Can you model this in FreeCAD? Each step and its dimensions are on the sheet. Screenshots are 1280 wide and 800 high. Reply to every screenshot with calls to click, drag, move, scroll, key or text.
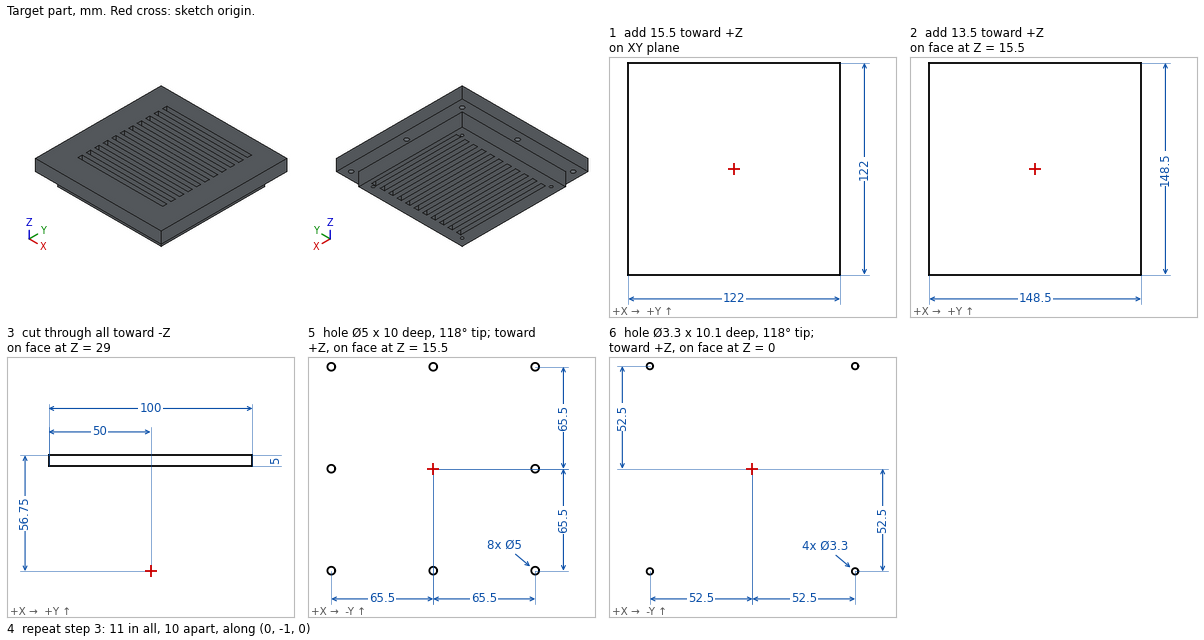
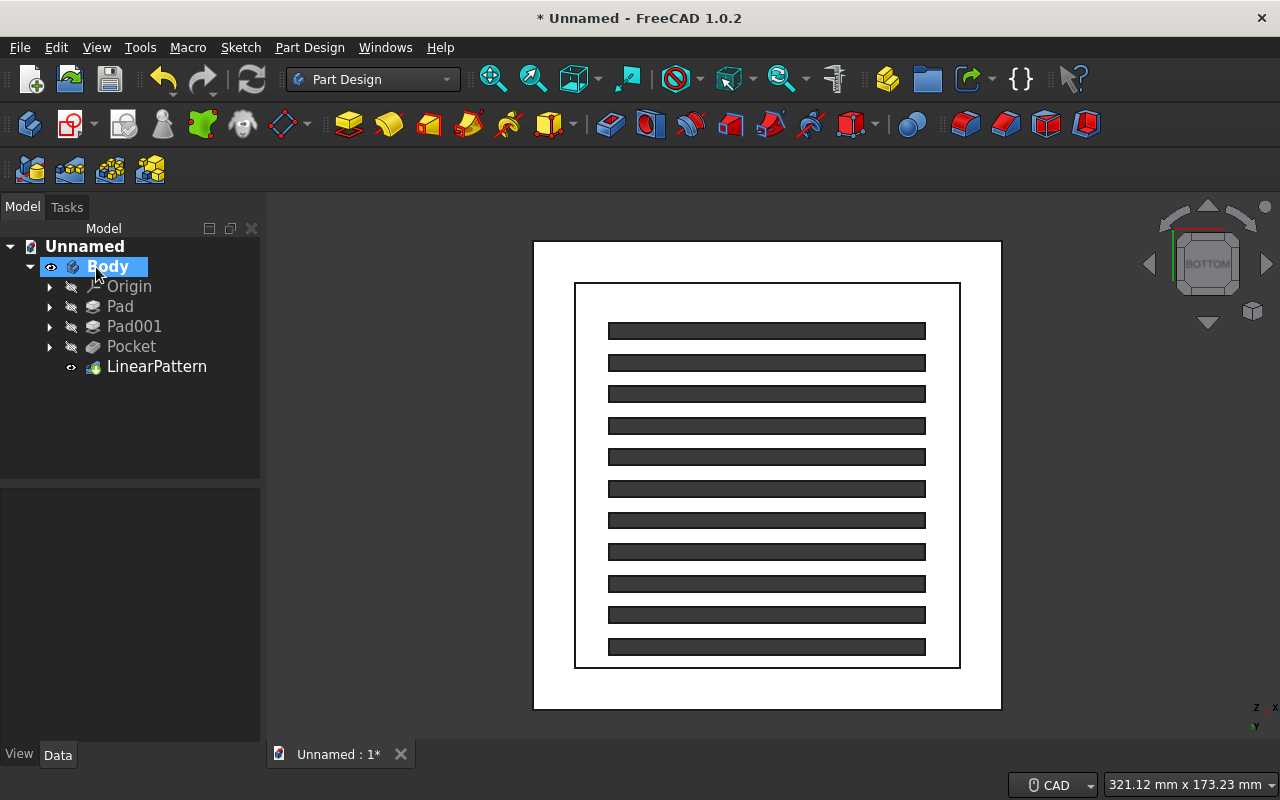
click(968, 675)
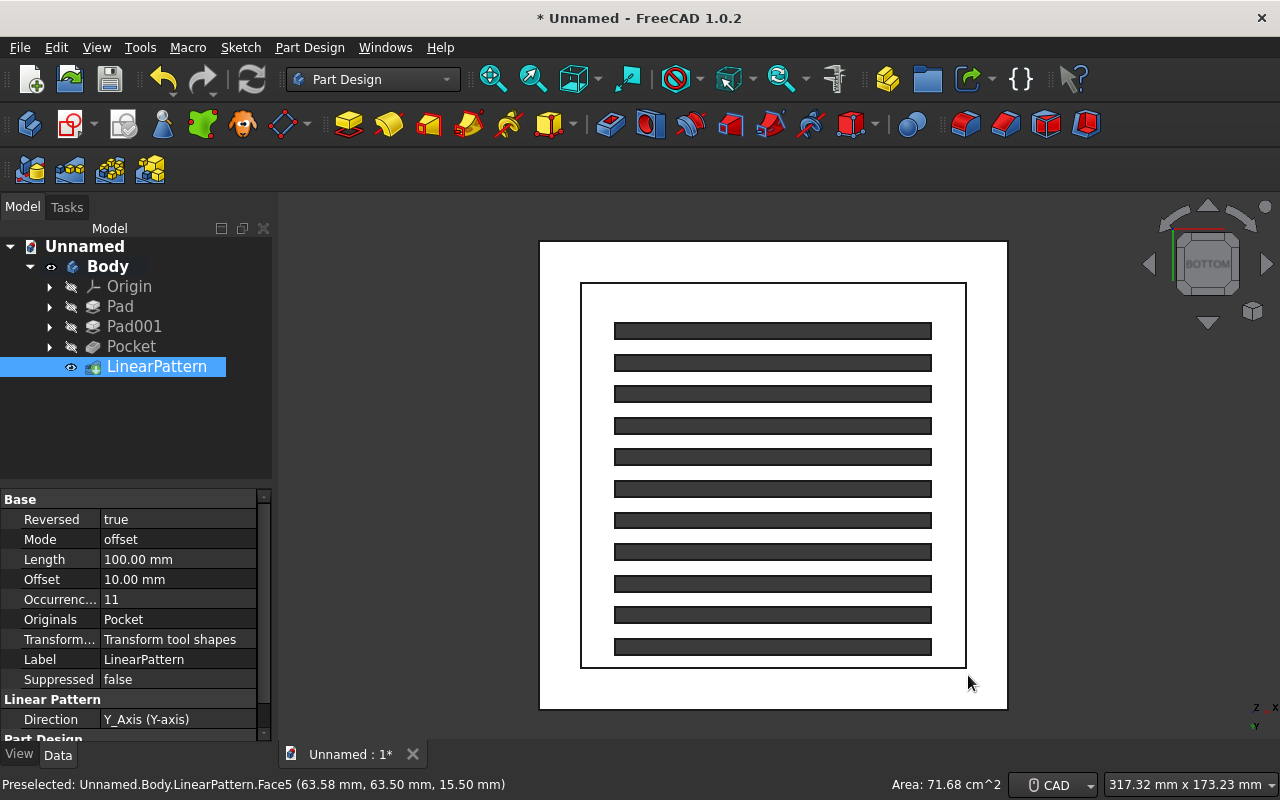
click(70, 124)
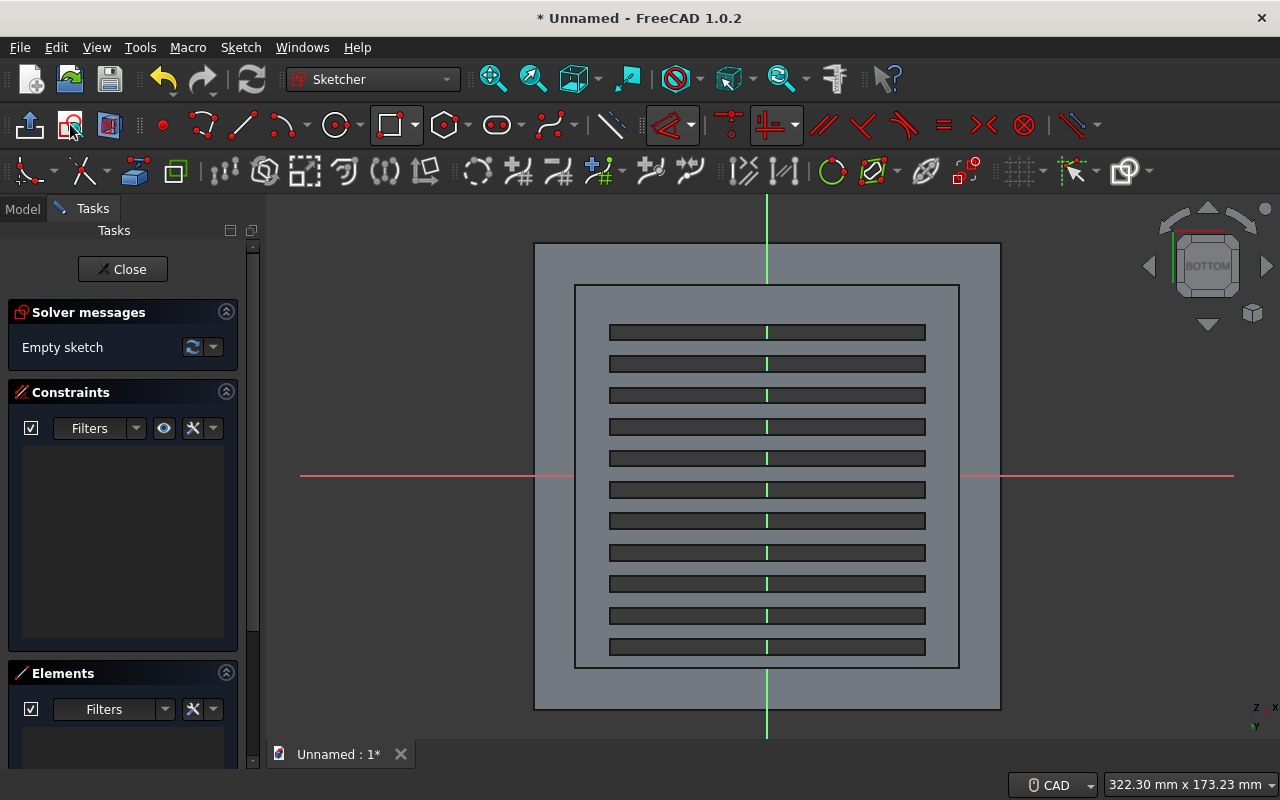
scroll(421, 422, down, 1)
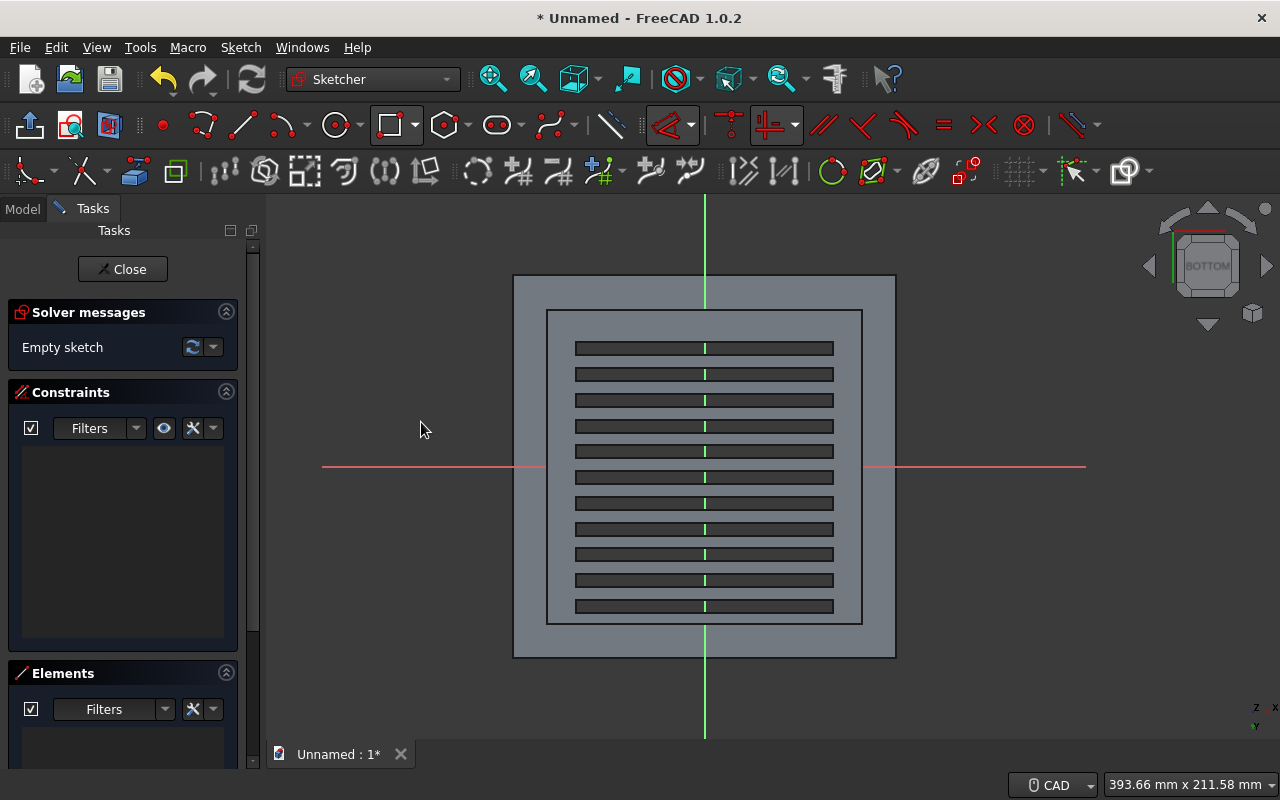
click(336, 126)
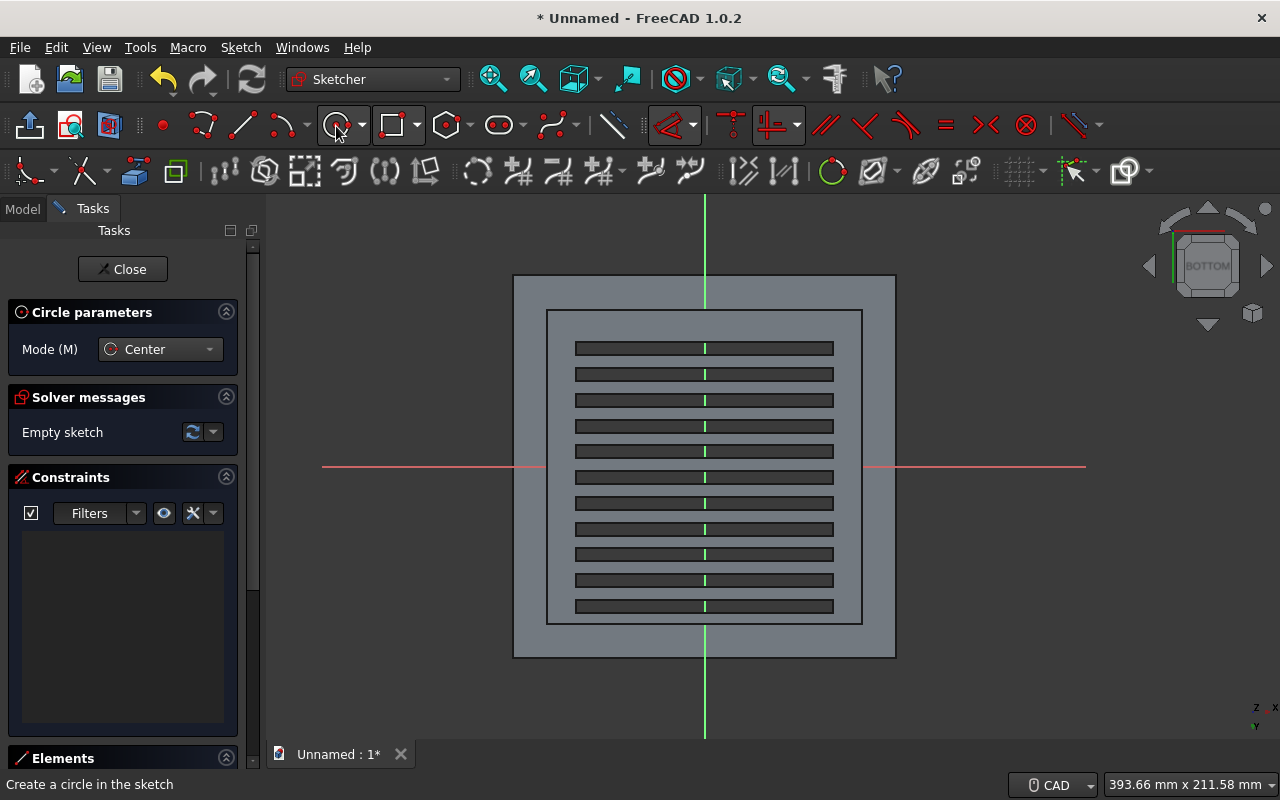
scroll(873, 635, up, 7)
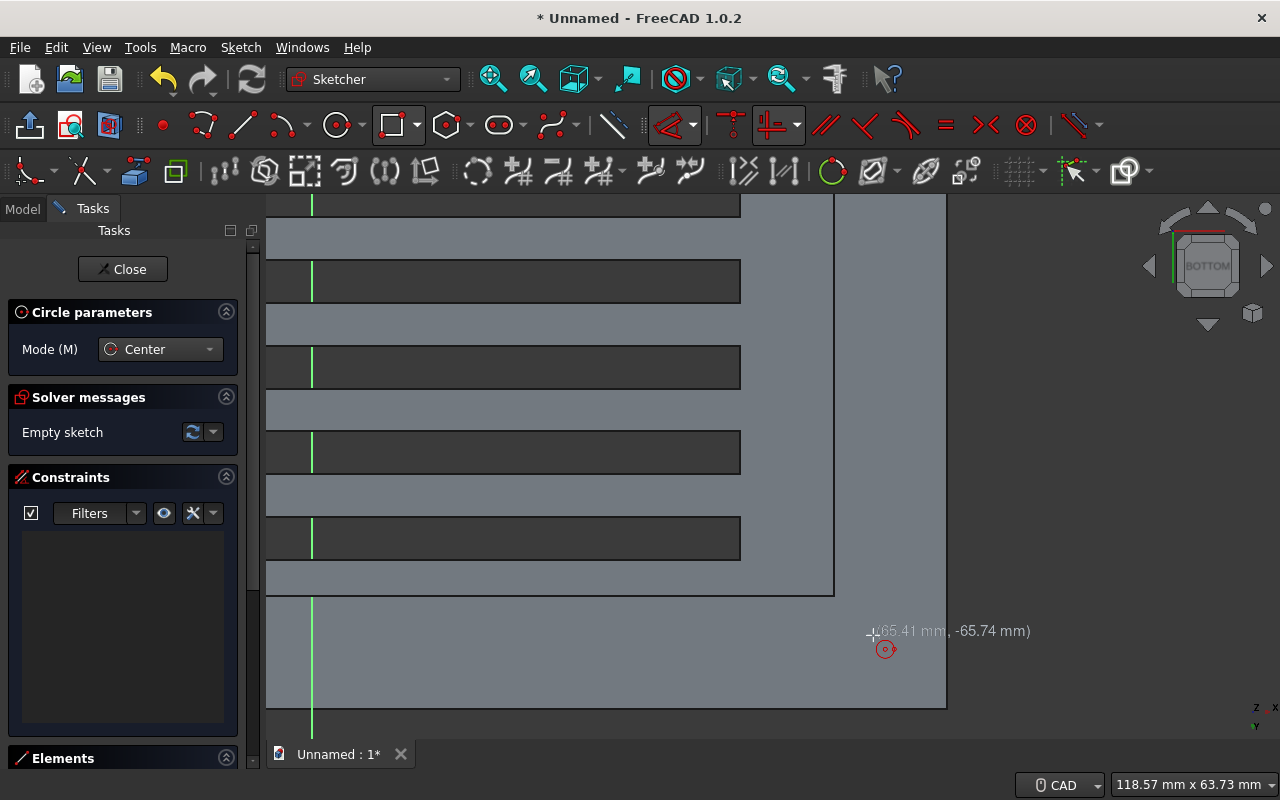
scroll(874, 636, down, 7)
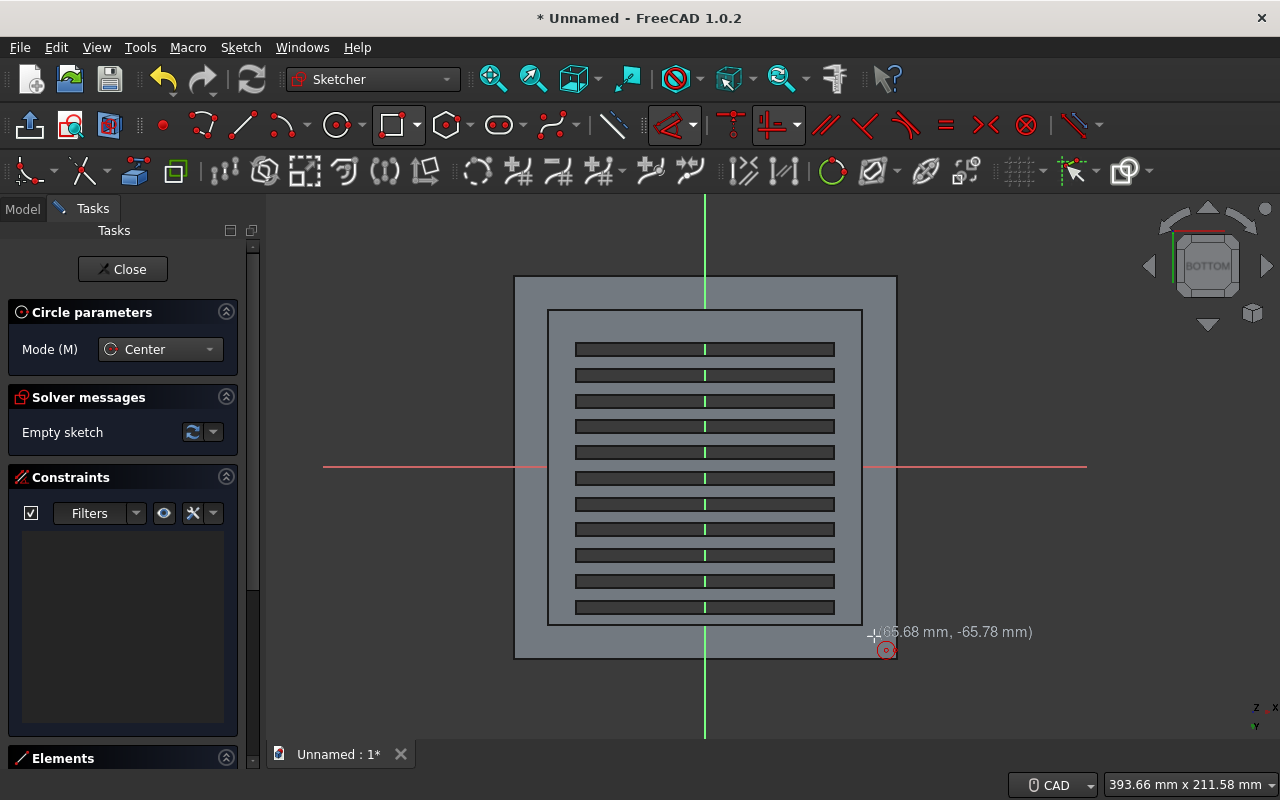
click(874, 636)
move(879, 632)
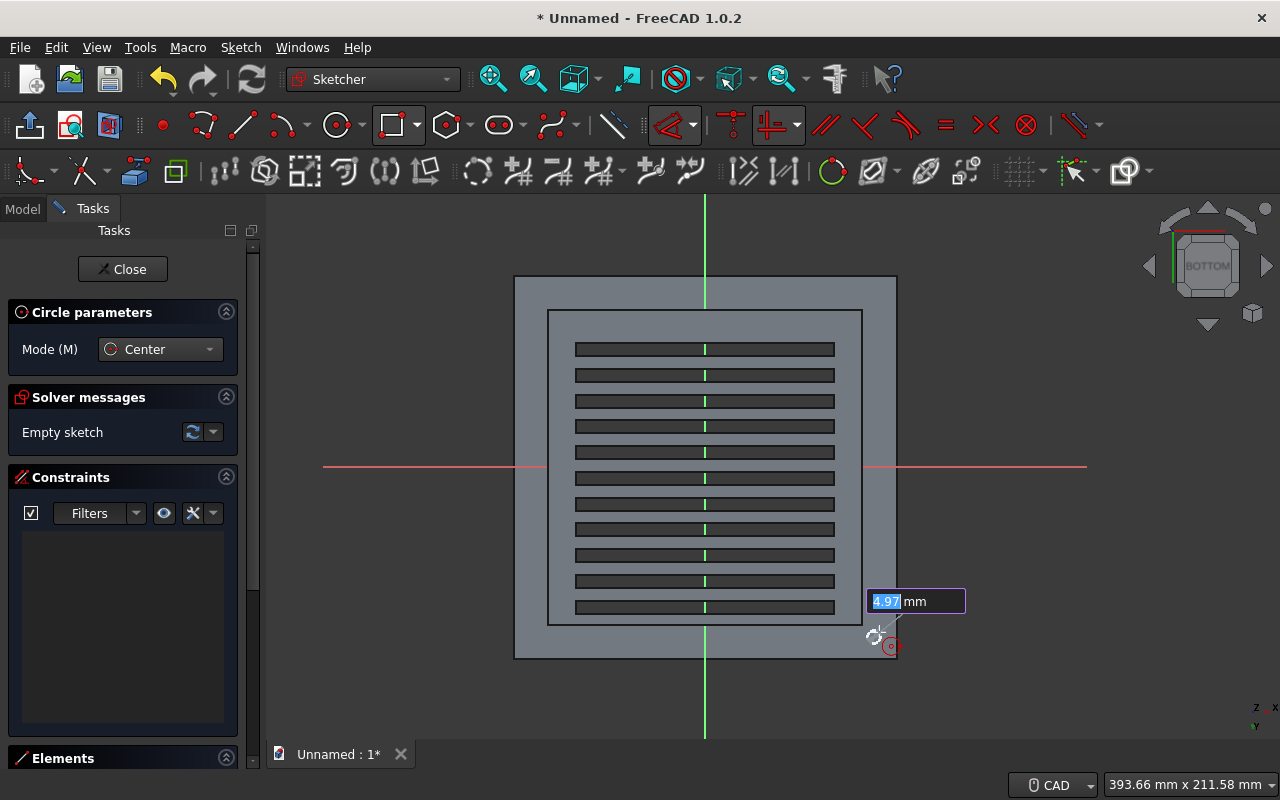
text(5)
key(Return)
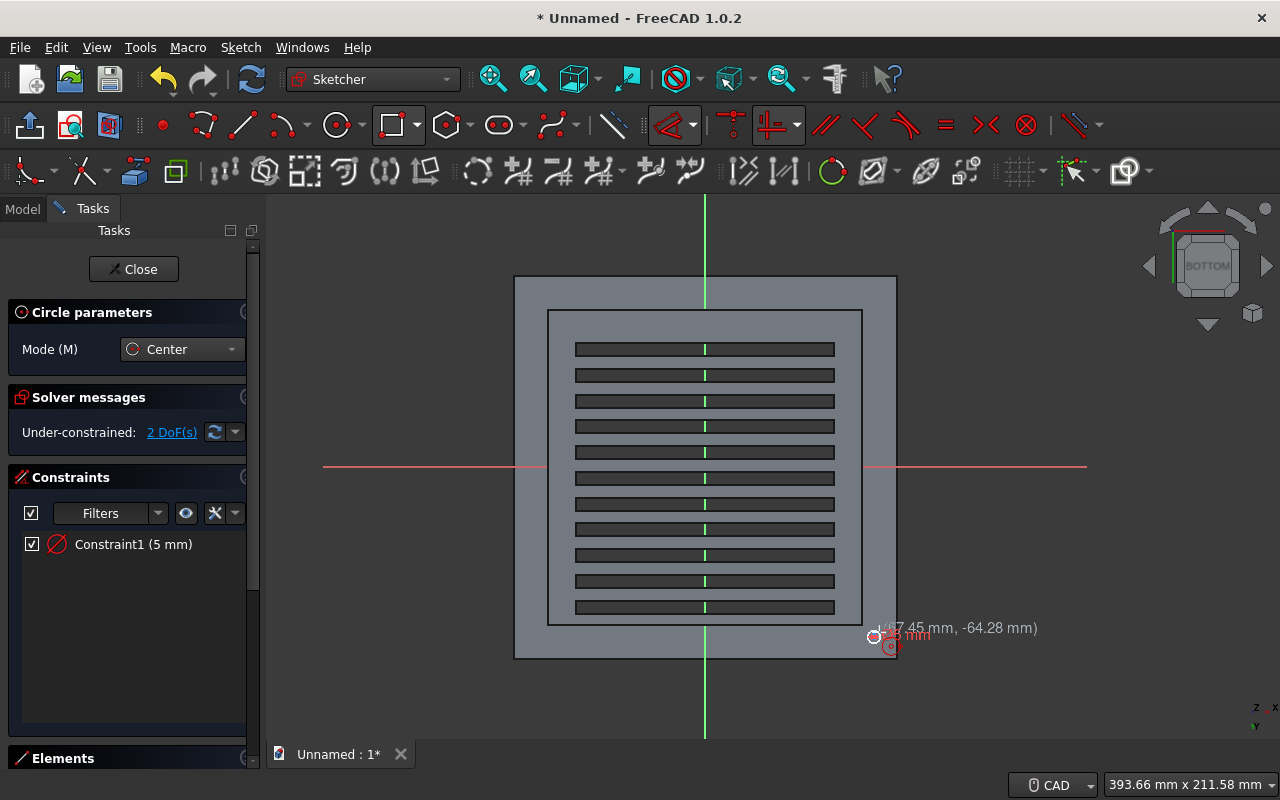
scroll(705, 636, up, 7)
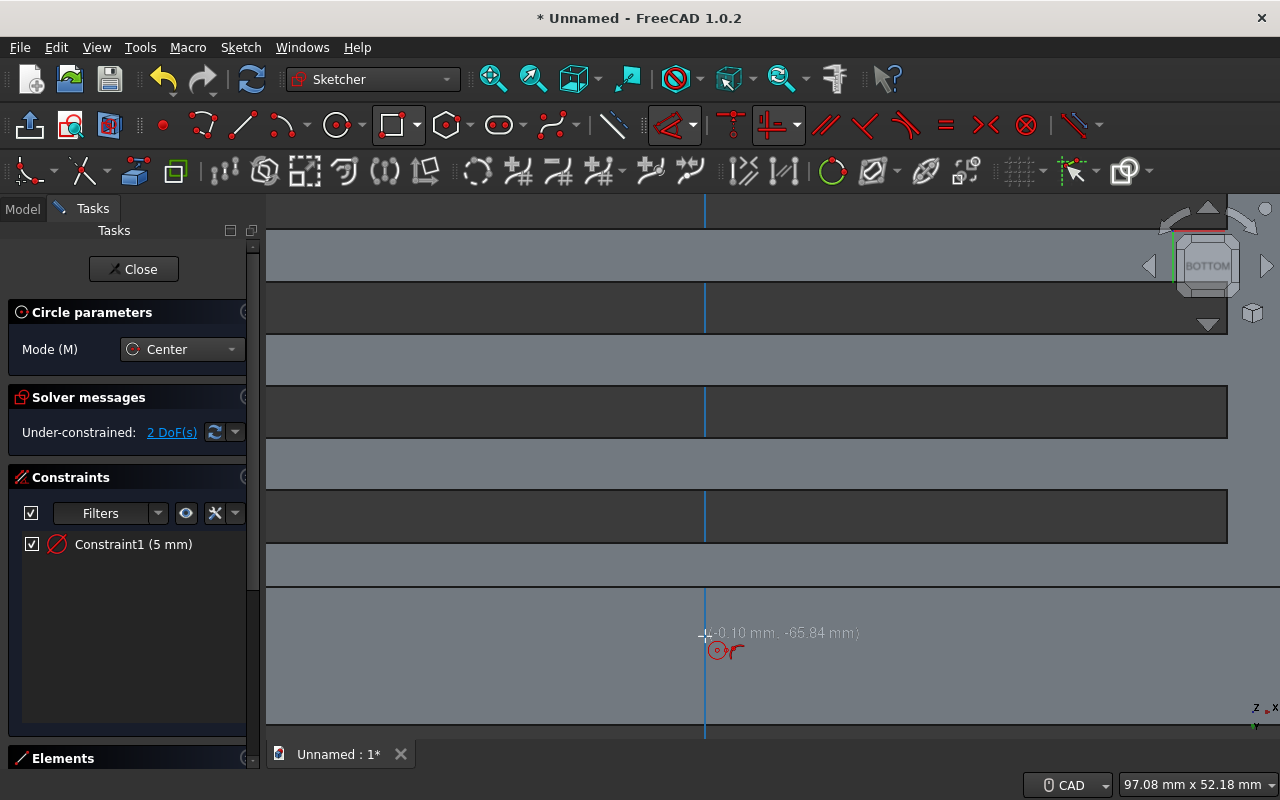
scroll(704, 636, down, 7)